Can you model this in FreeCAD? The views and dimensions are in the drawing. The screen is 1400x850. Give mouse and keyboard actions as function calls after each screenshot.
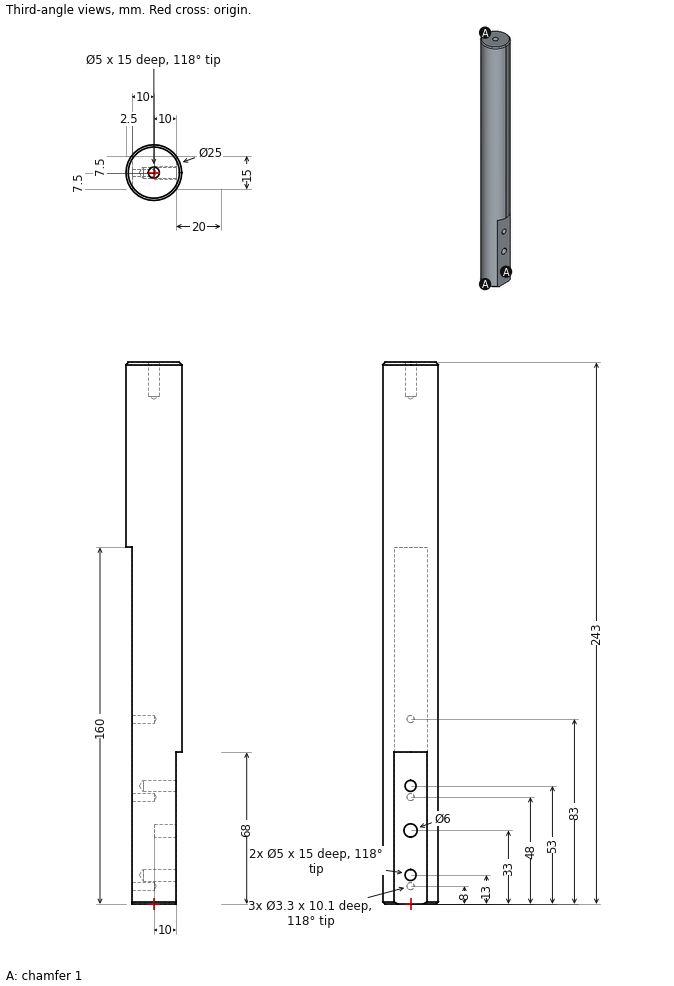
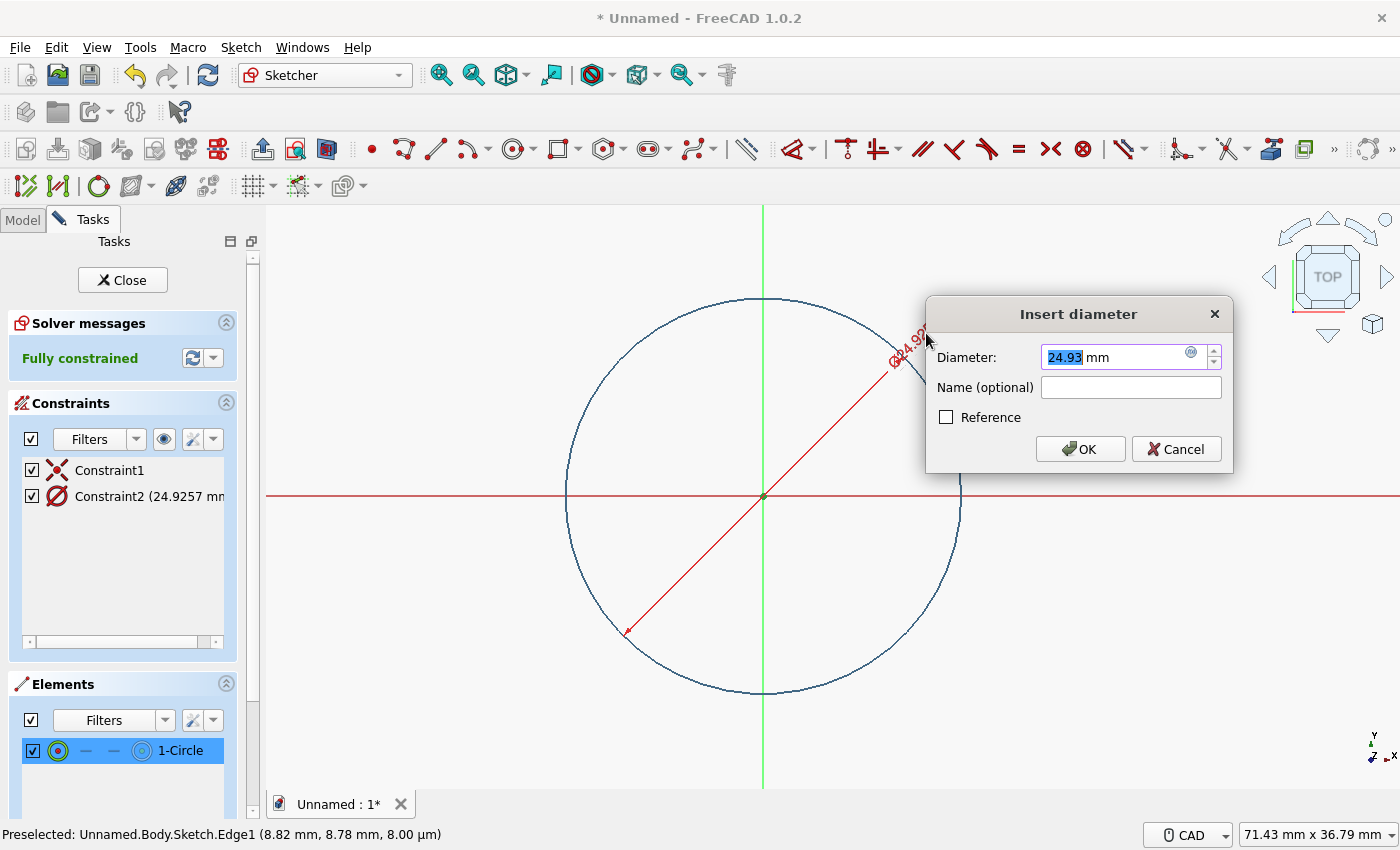
text(25)
key(Return)
key(Escape)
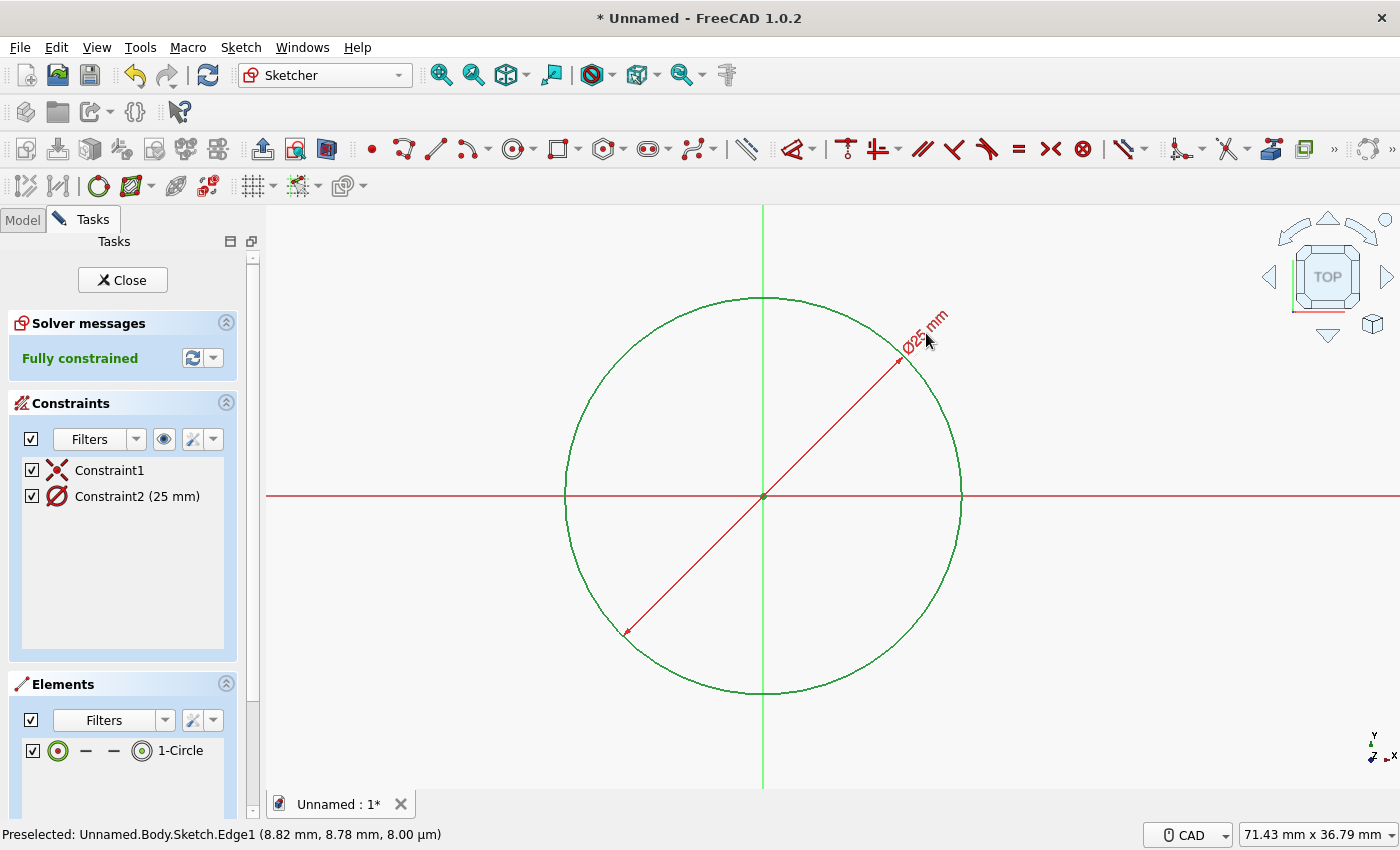
click(123, 280)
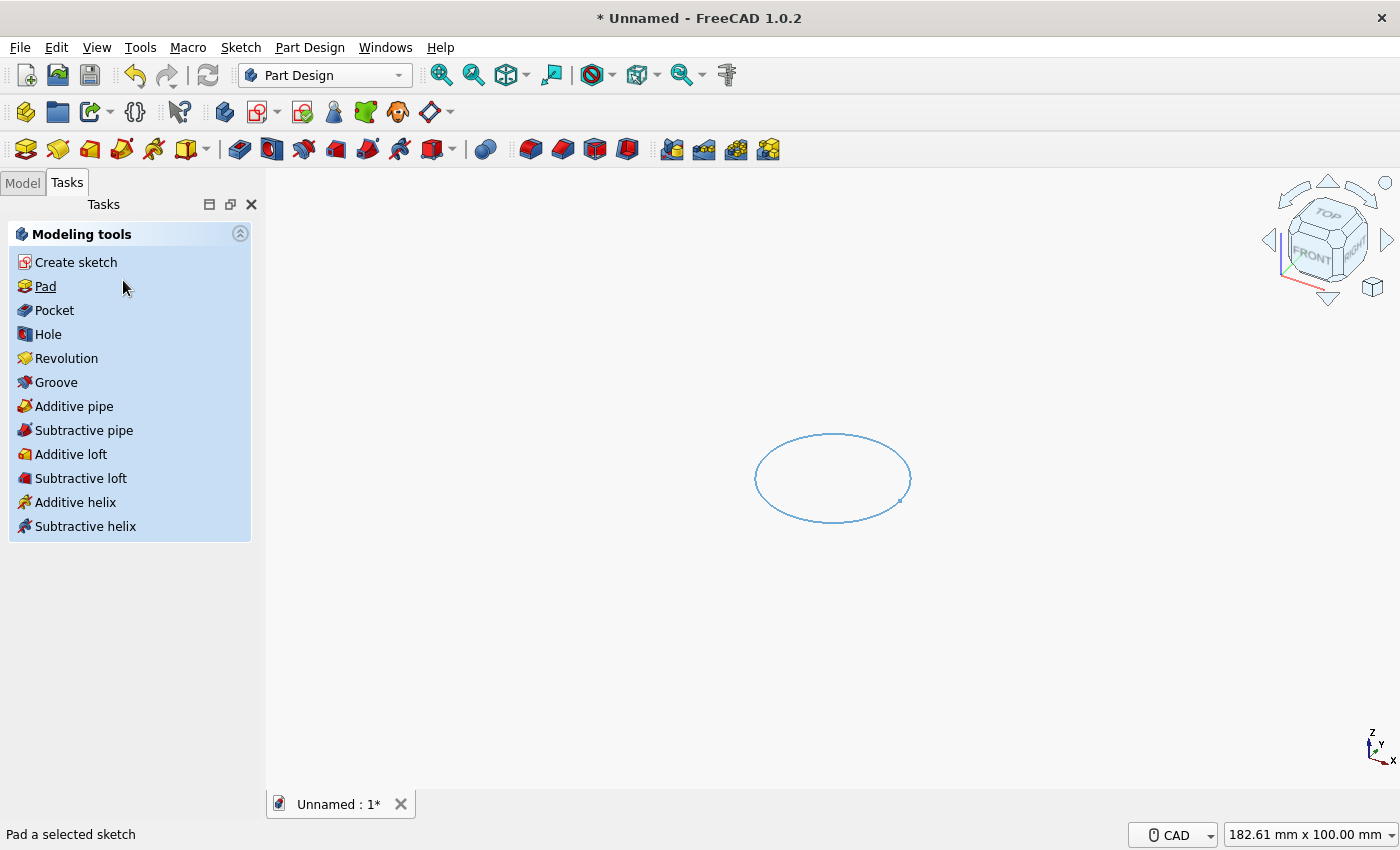
click(26, 150)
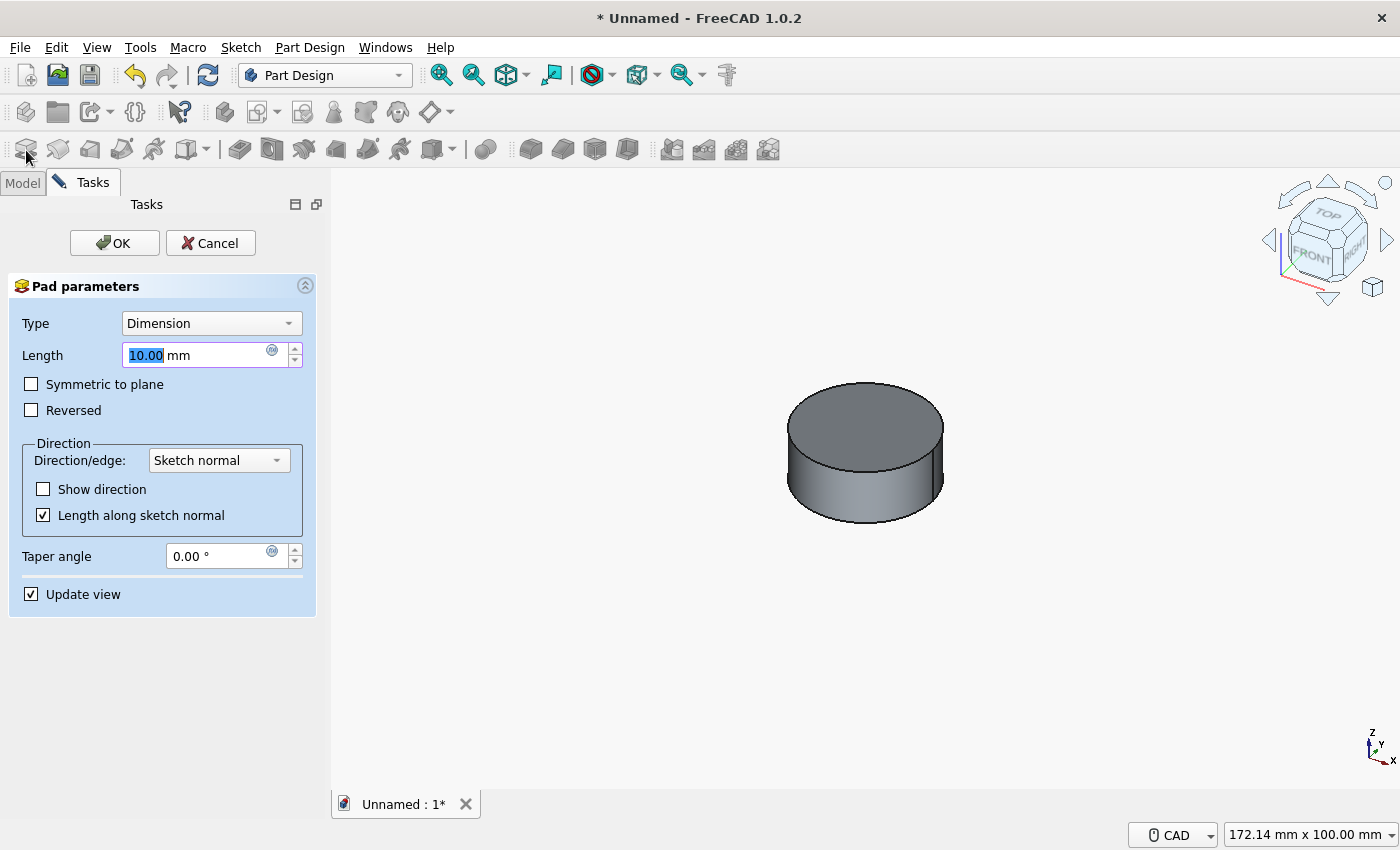
text(243)
key(Tab)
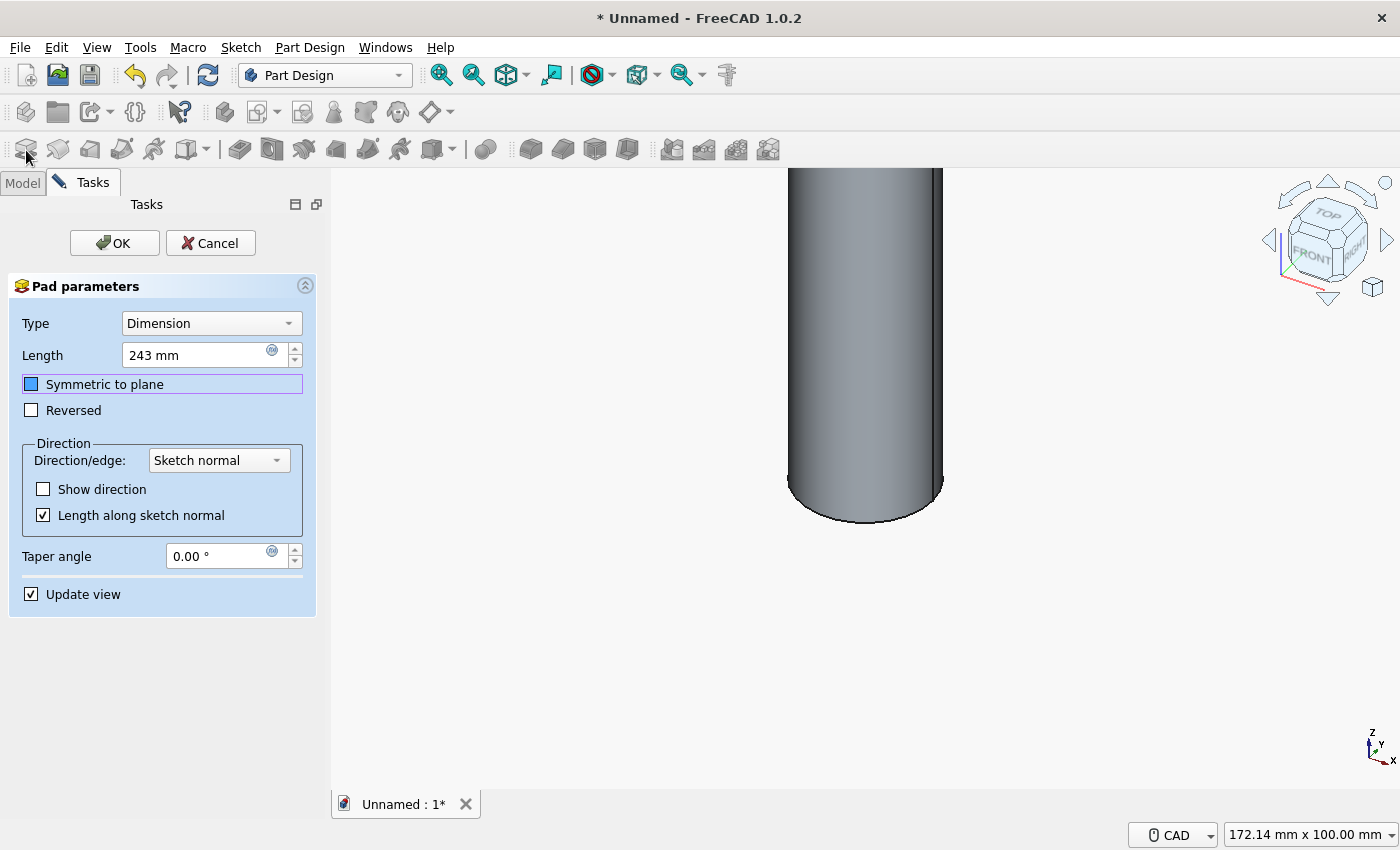
click(115, 243)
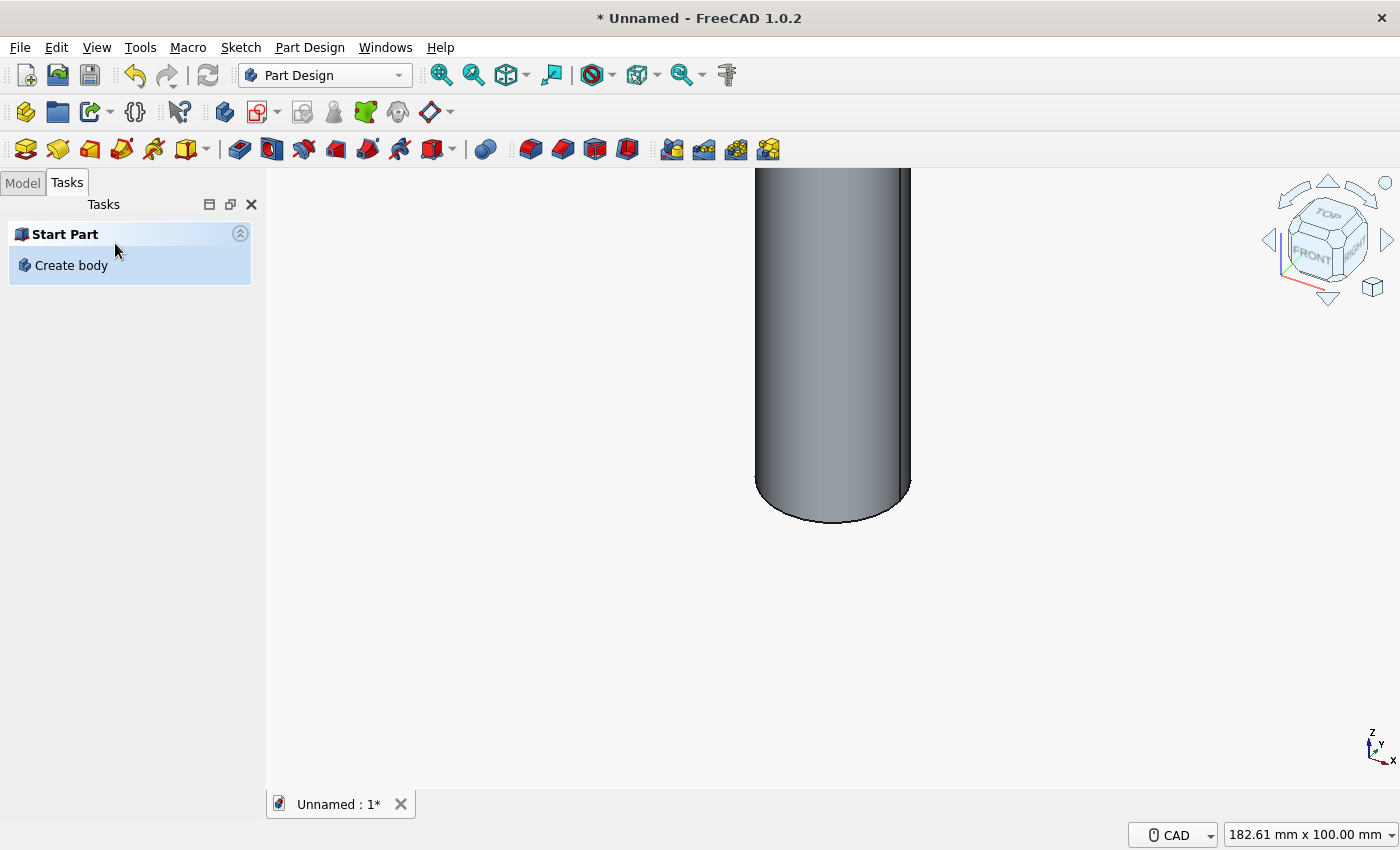
click(442, 76)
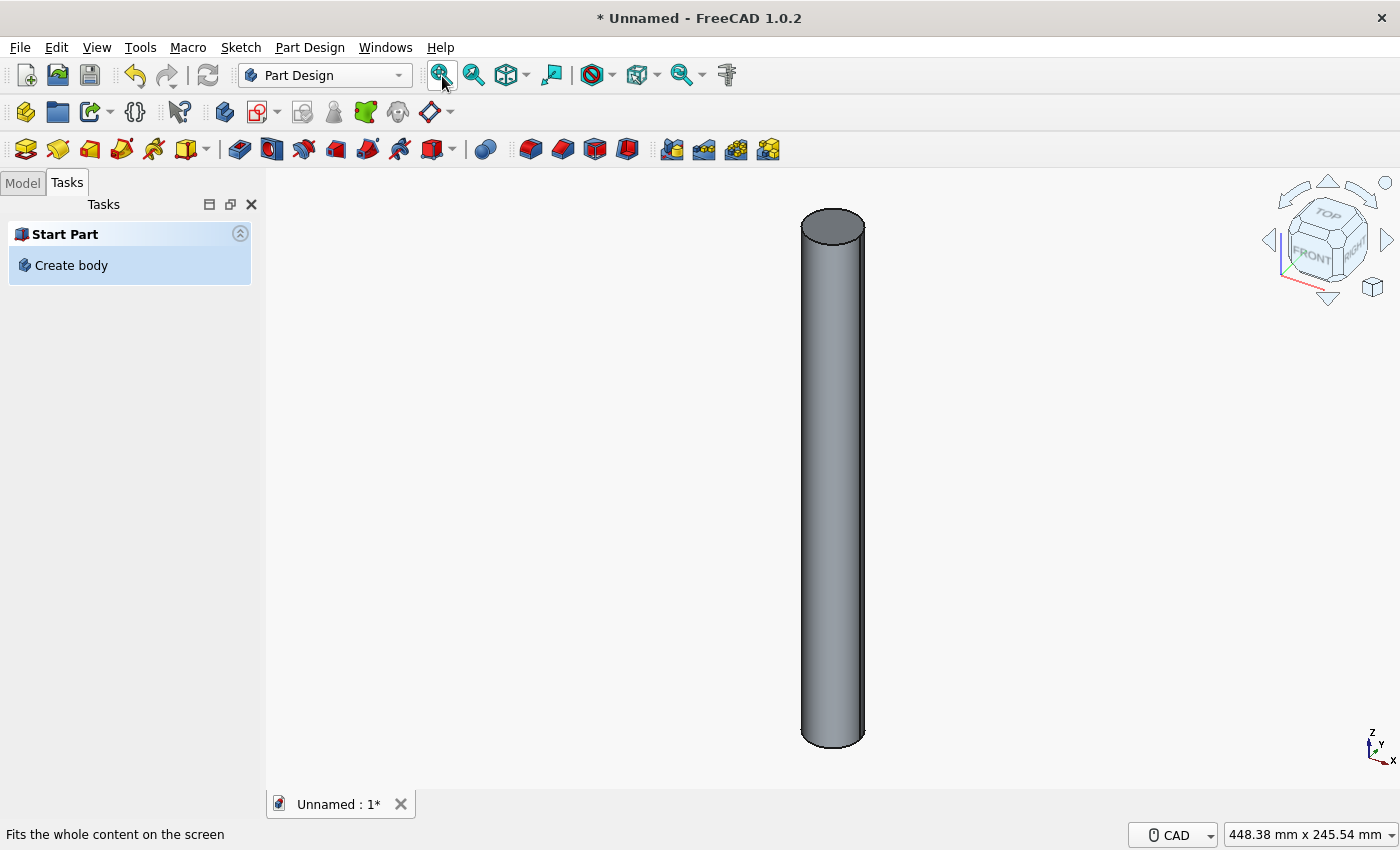
click(258, 112)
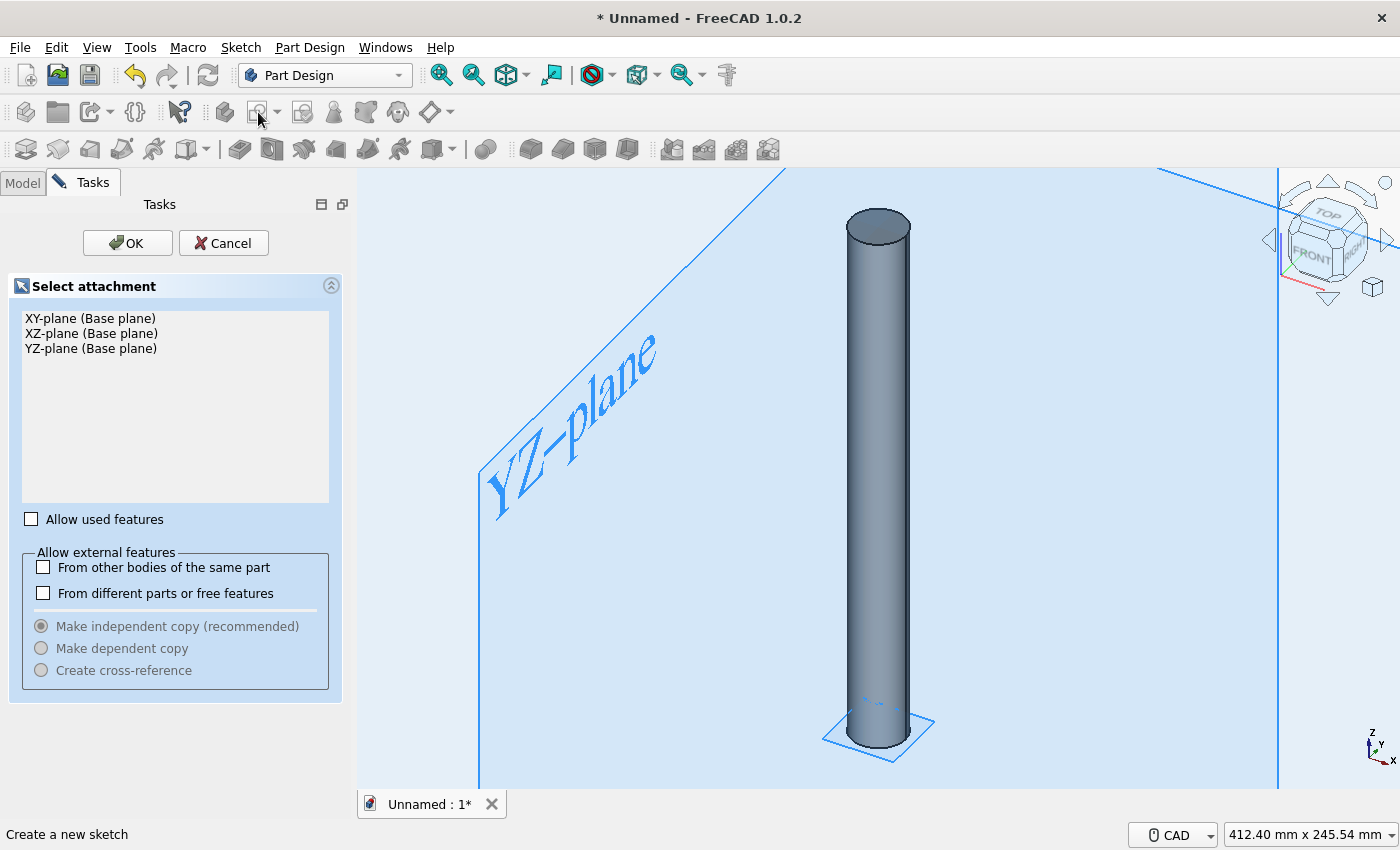
click(82, 318)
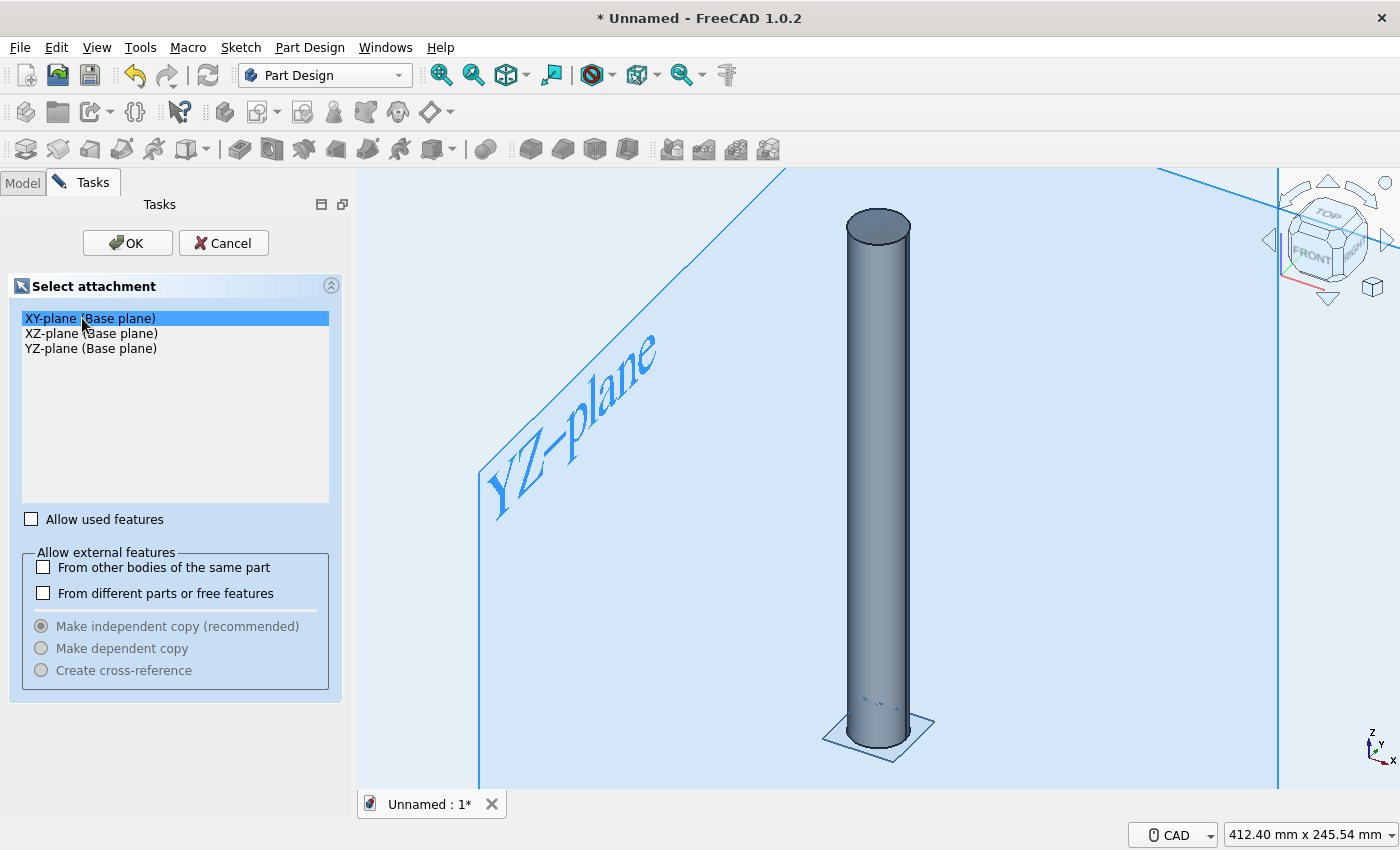
click(128, 243)